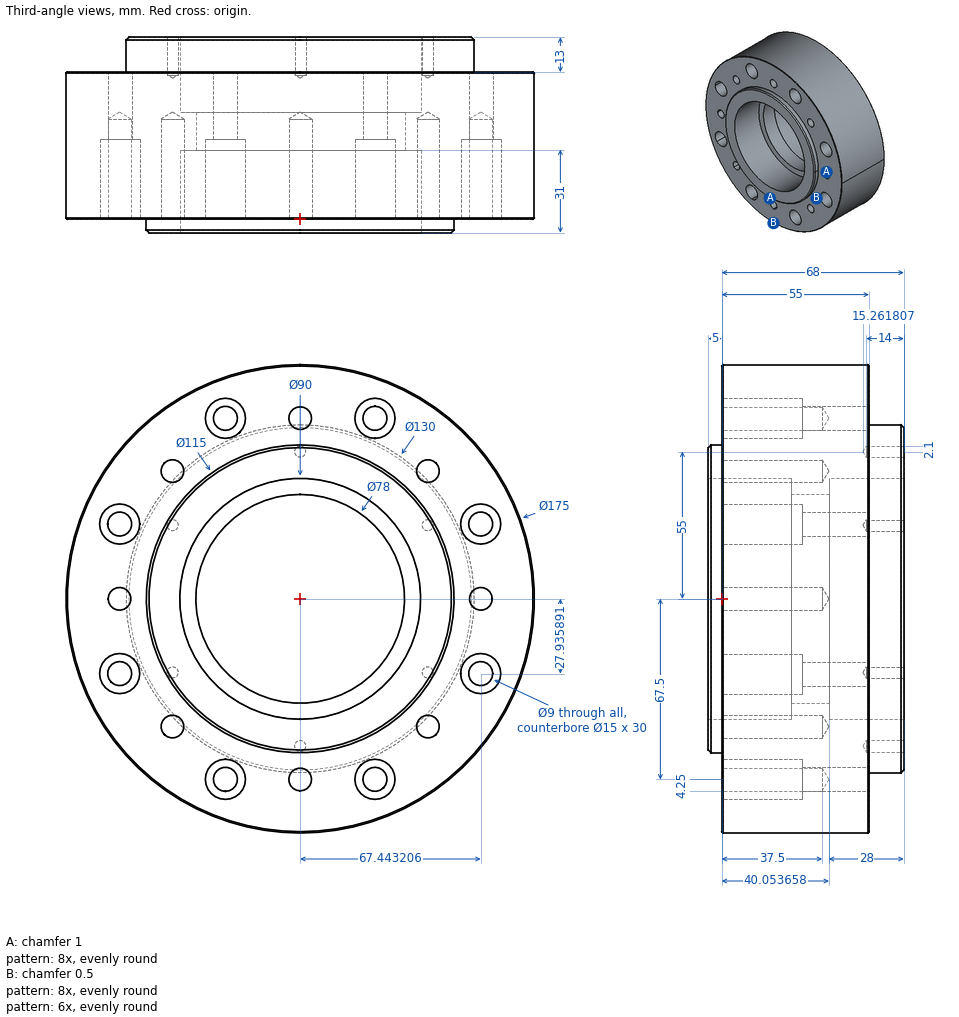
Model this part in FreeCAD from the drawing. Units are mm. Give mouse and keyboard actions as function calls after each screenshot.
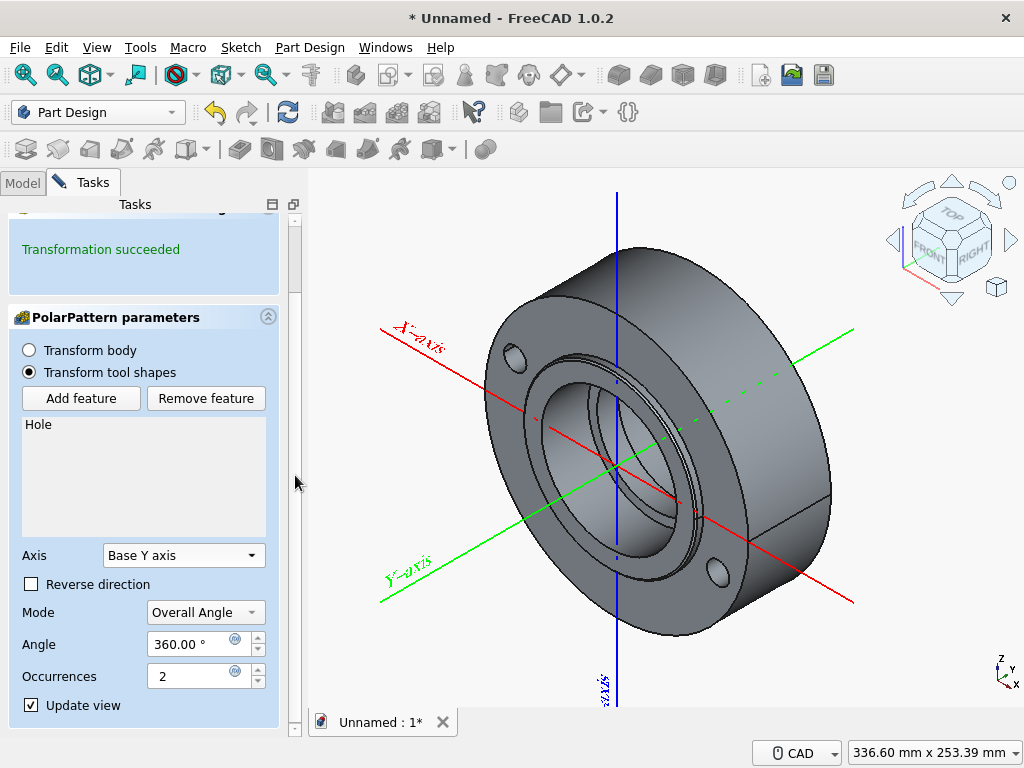
triple_click(198, 676)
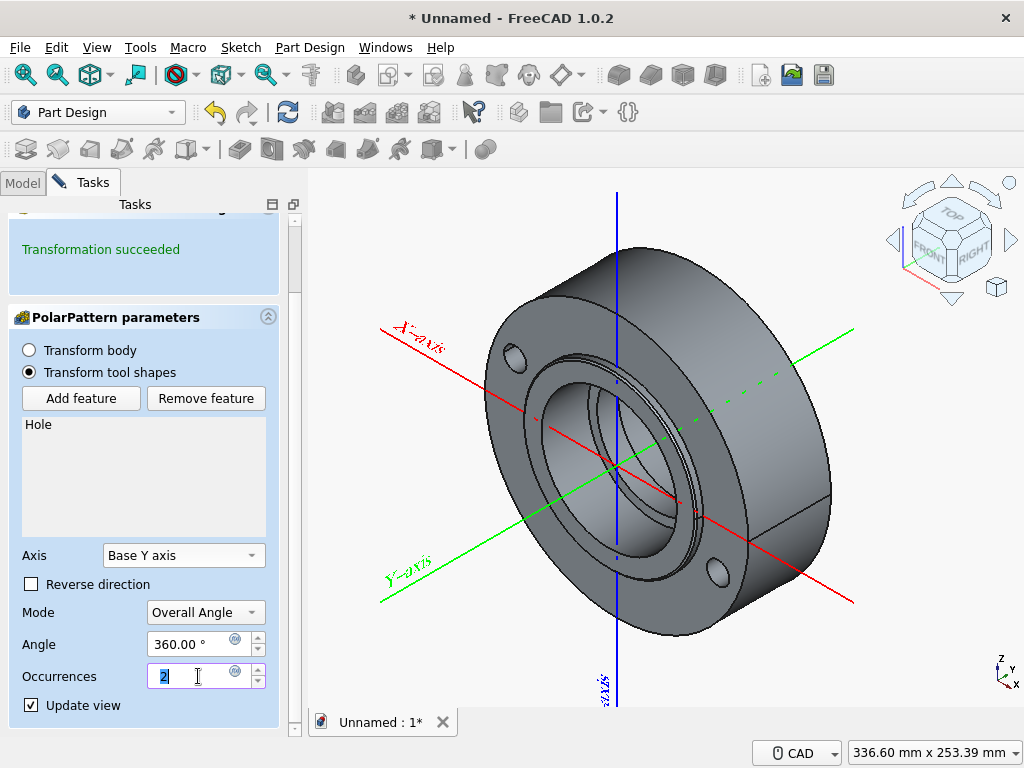
text(8)
key(Tab)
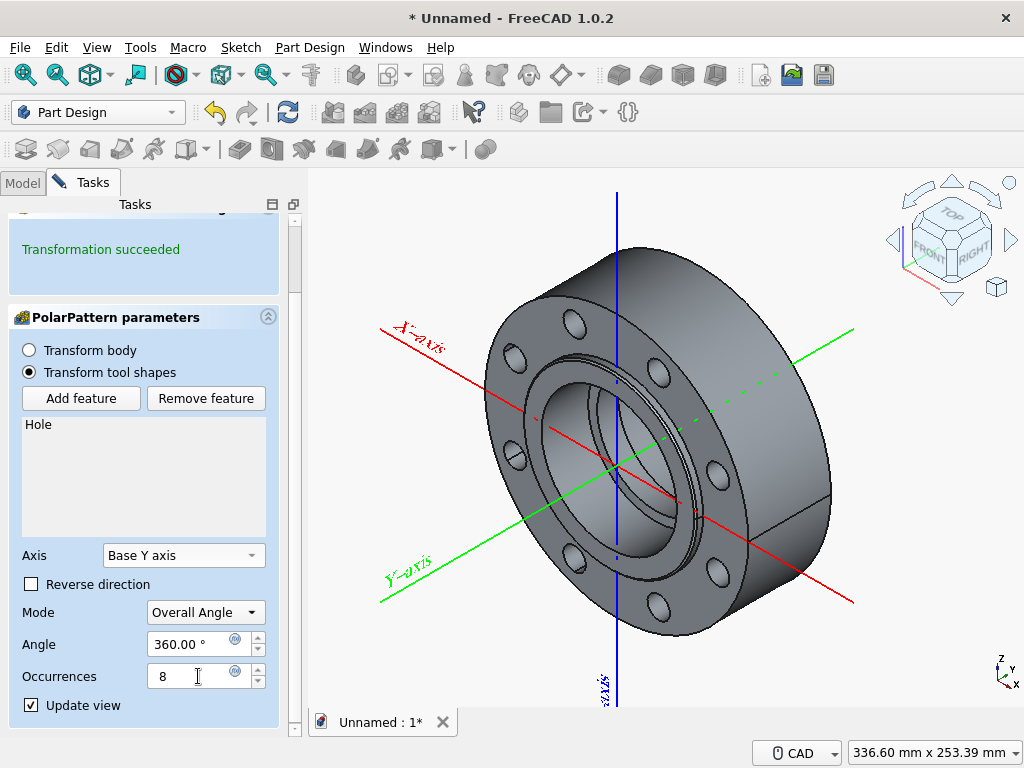
scroll(295, 475, up, 3)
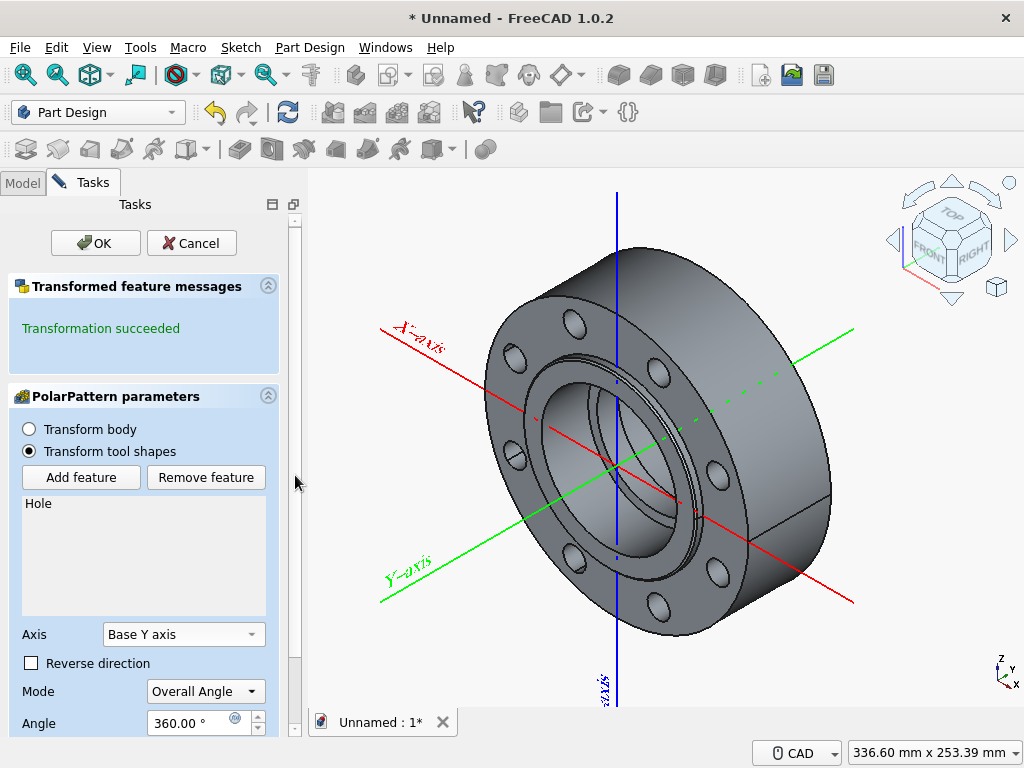
click(96, 243)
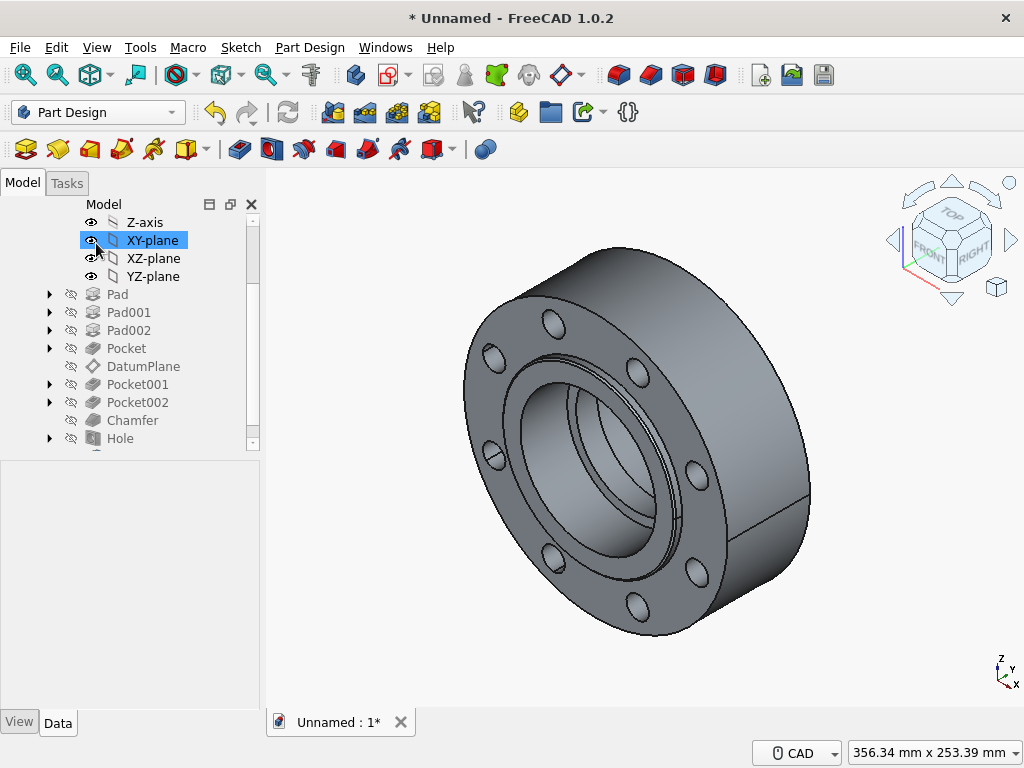
click(555, 297)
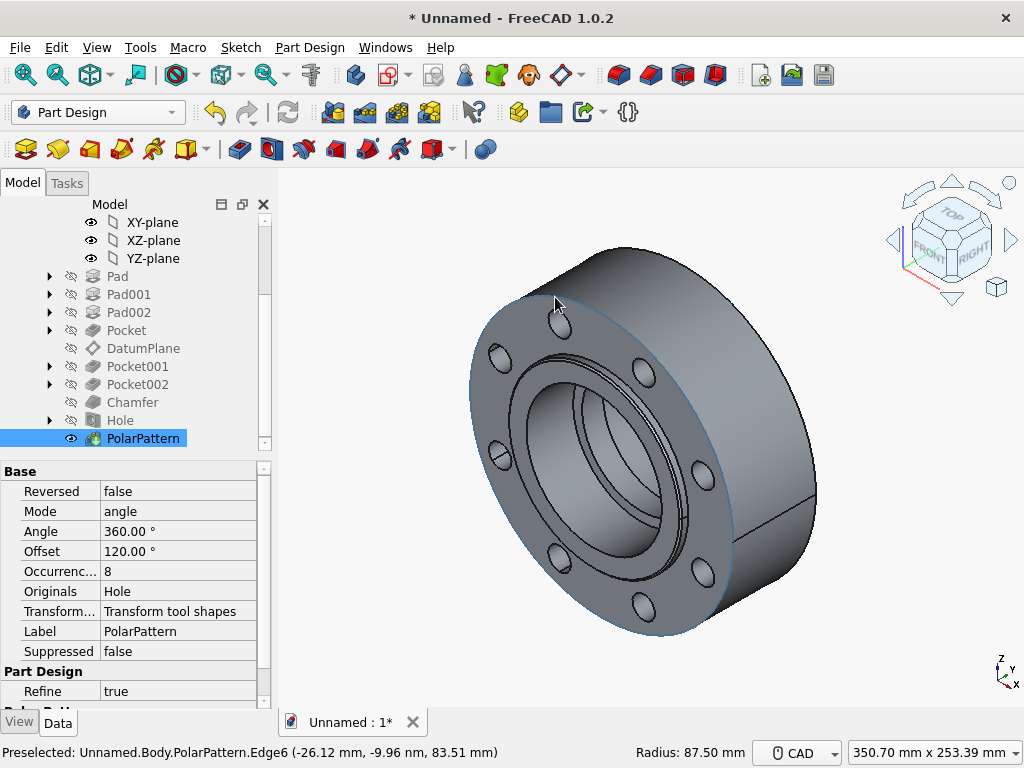
key(2)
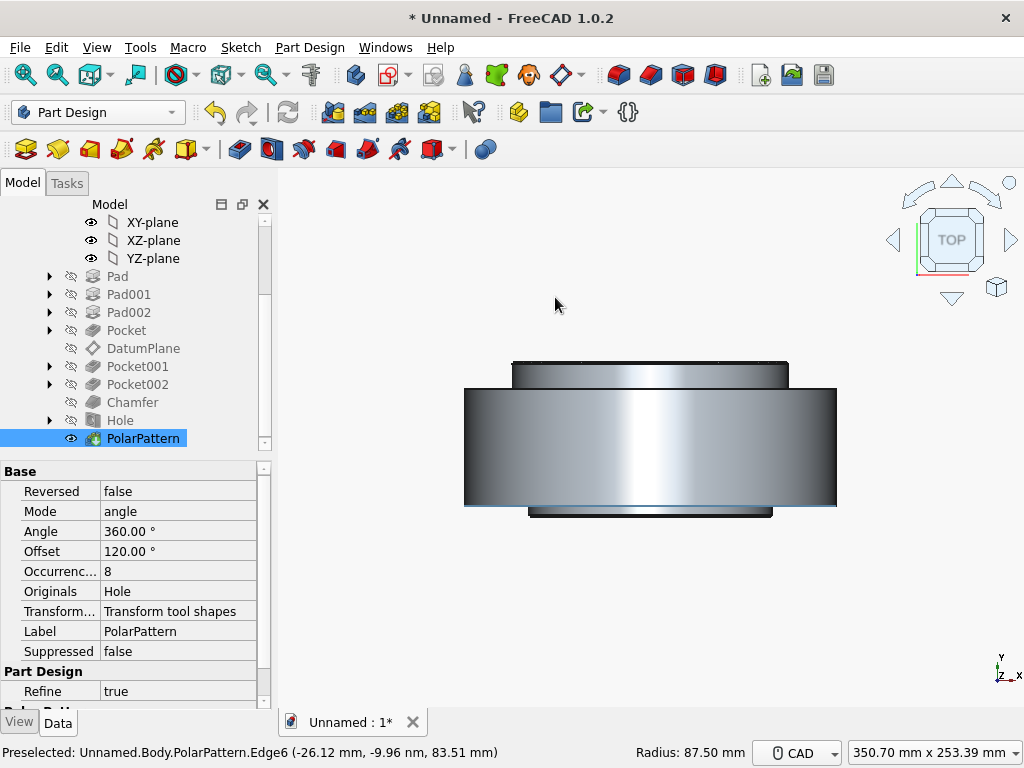
click(499, 388, ctrl)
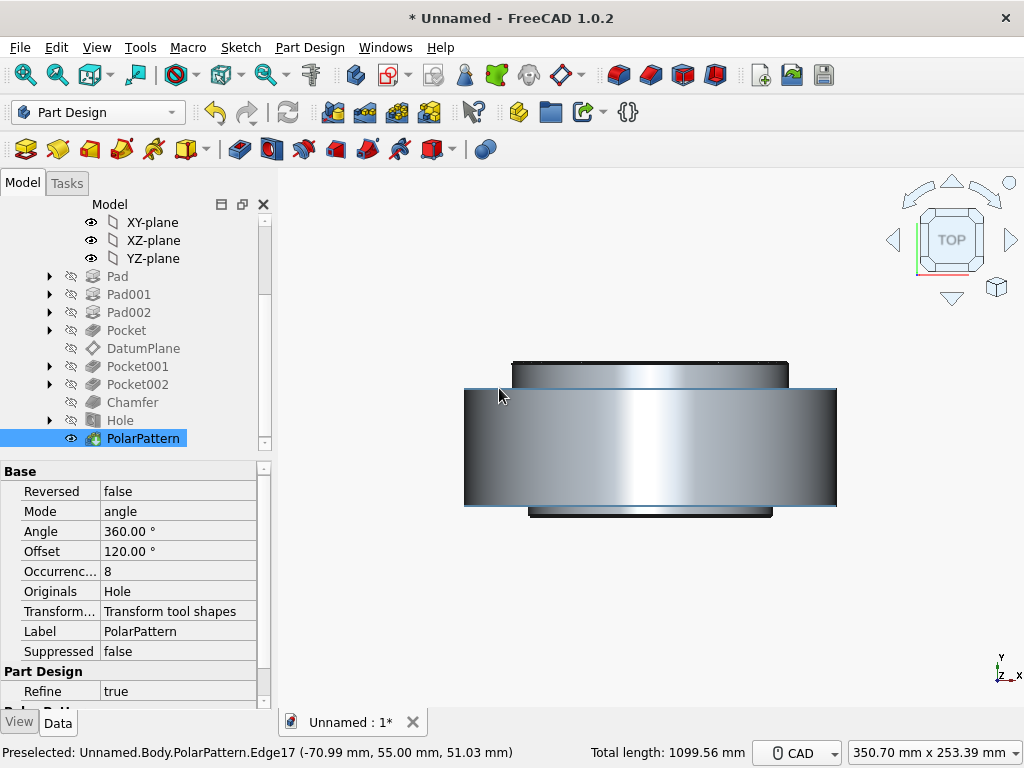
click(652, 76)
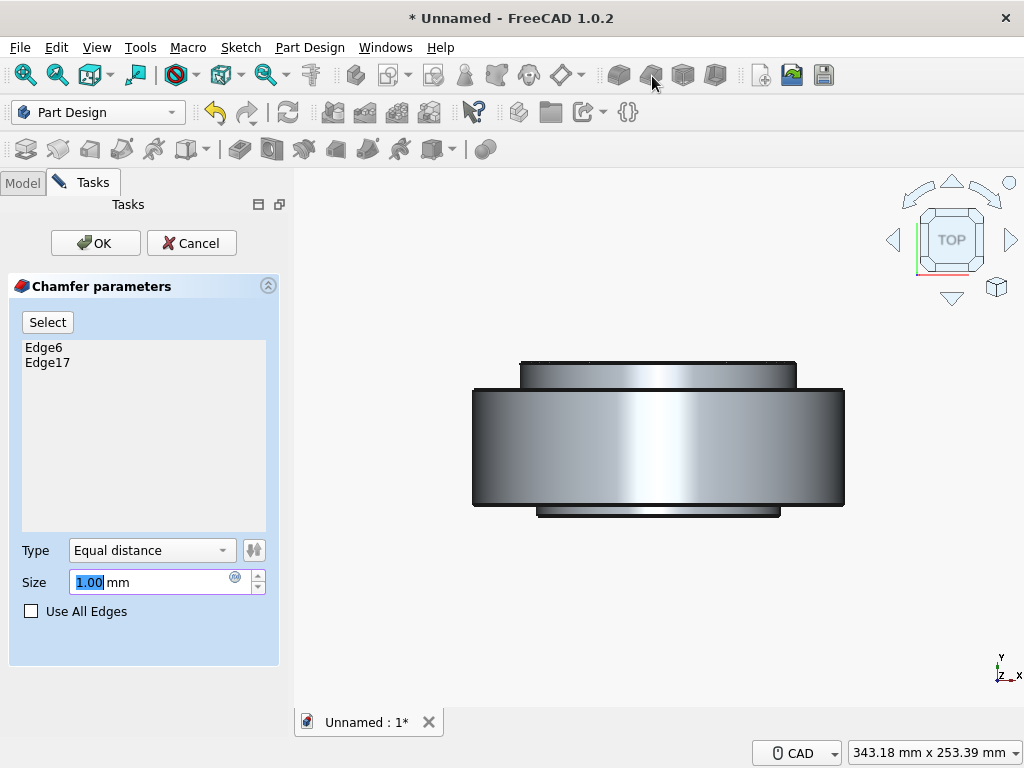
text(0.5)
key(Tab)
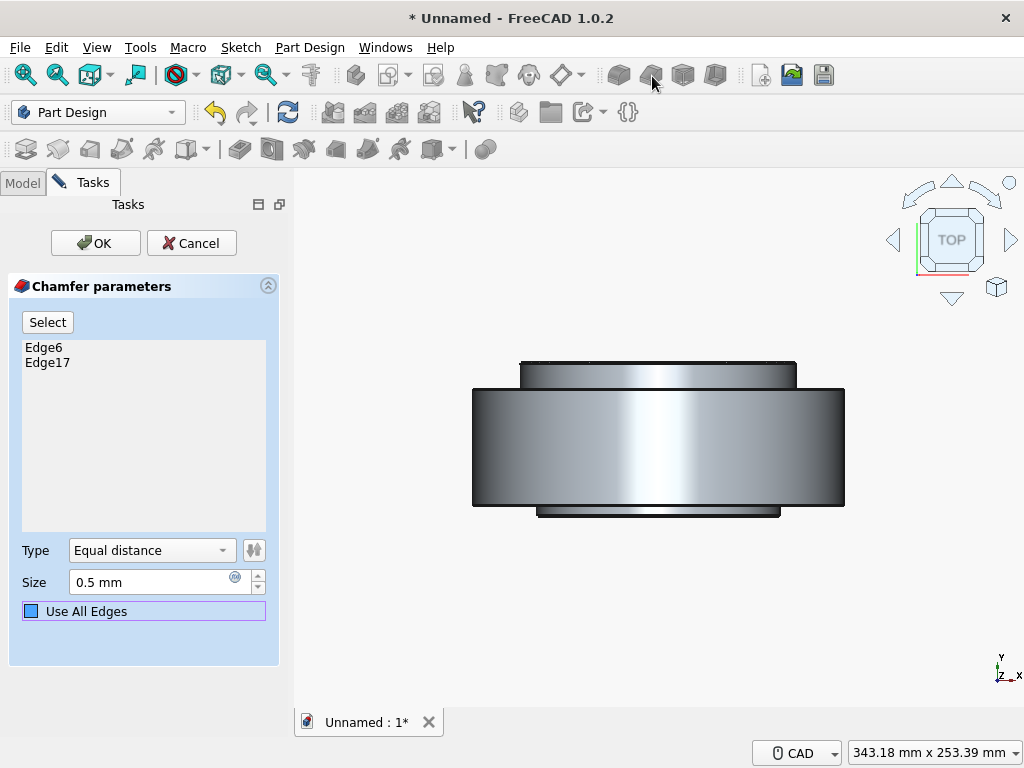
click(96, 243)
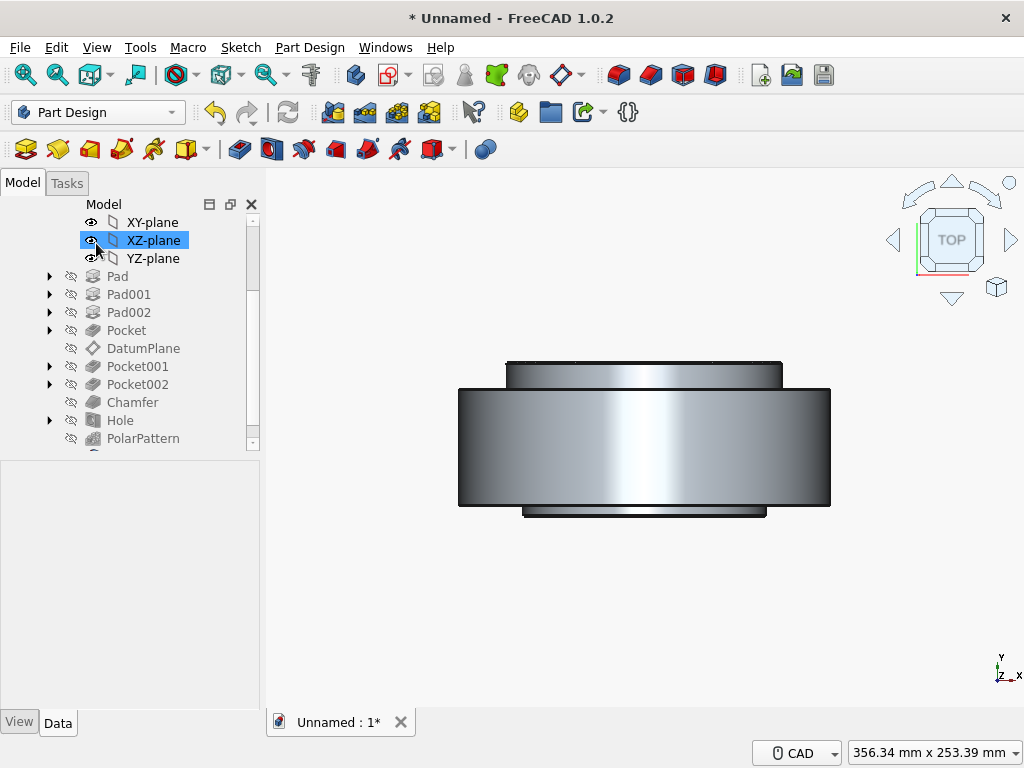
click(388, 76)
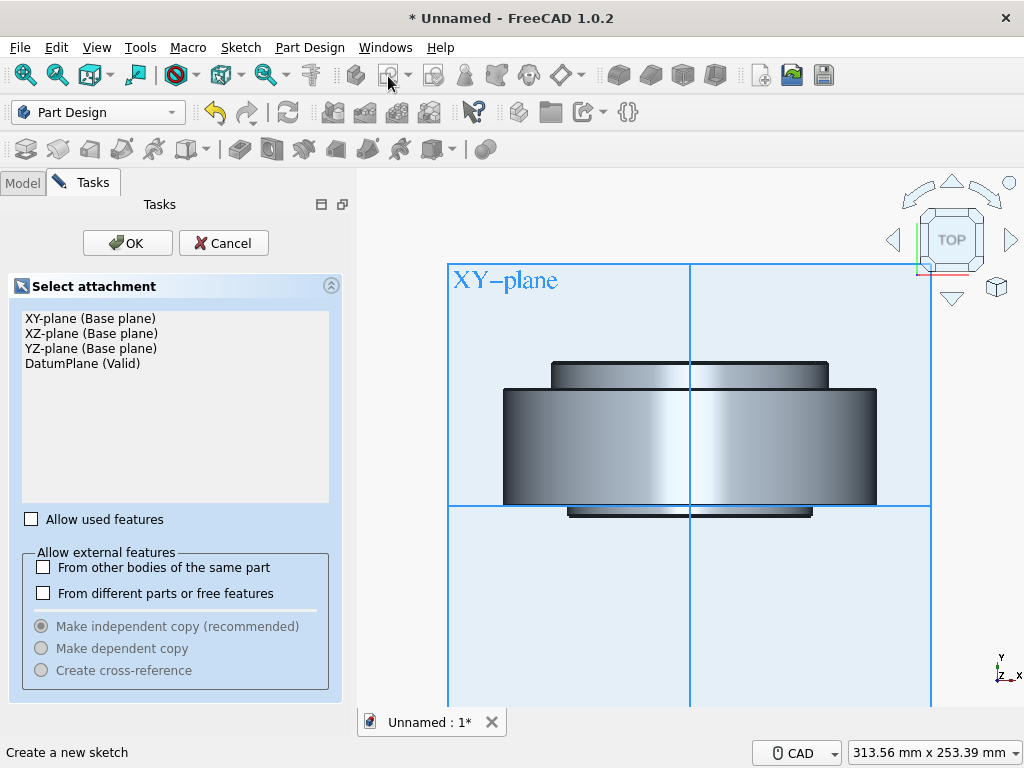
click(82, 348)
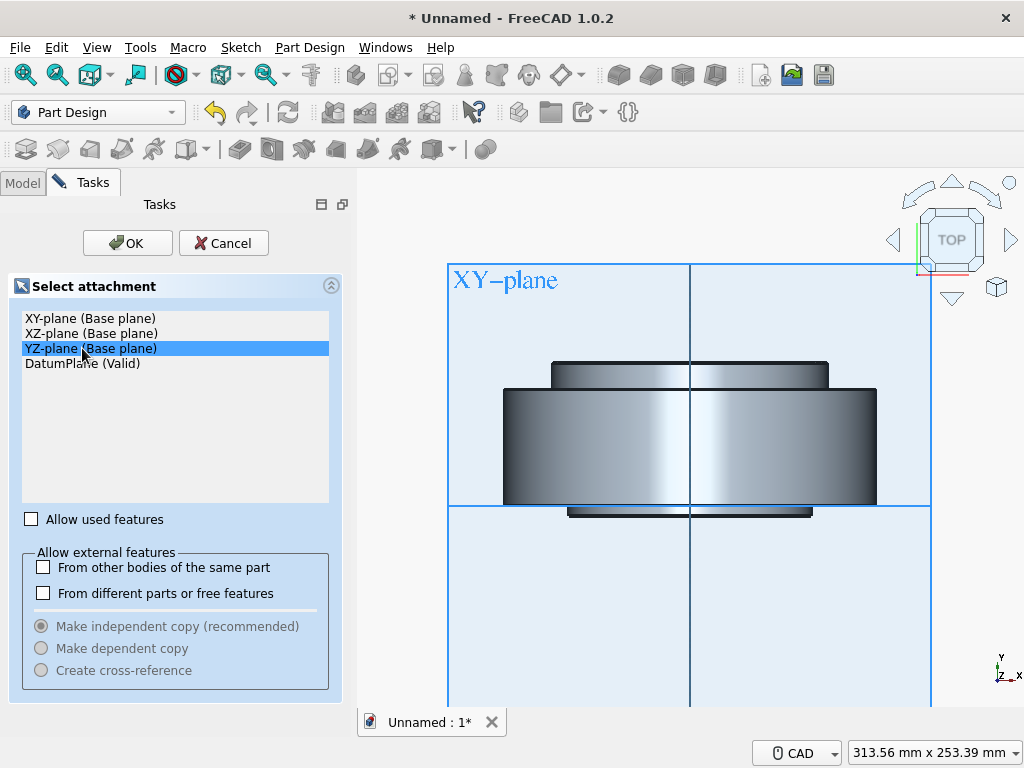
click(128, 243)